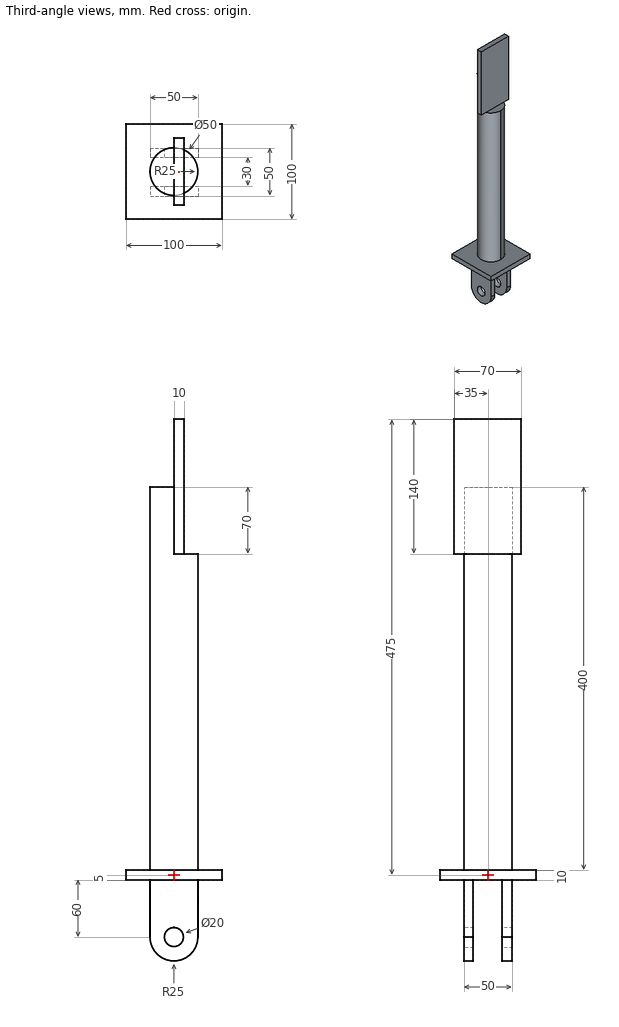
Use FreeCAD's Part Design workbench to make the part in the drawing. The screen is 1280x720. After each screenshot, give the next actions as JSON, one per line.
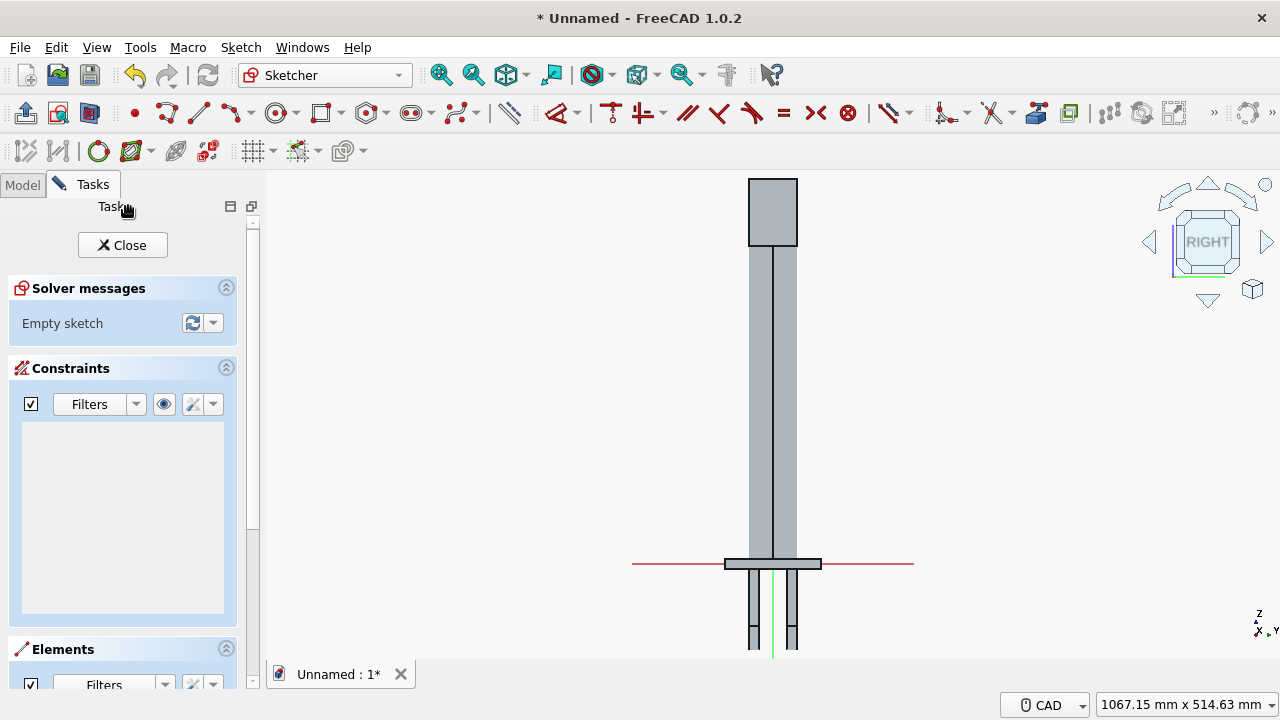
{"action": "key", "text": "q s"}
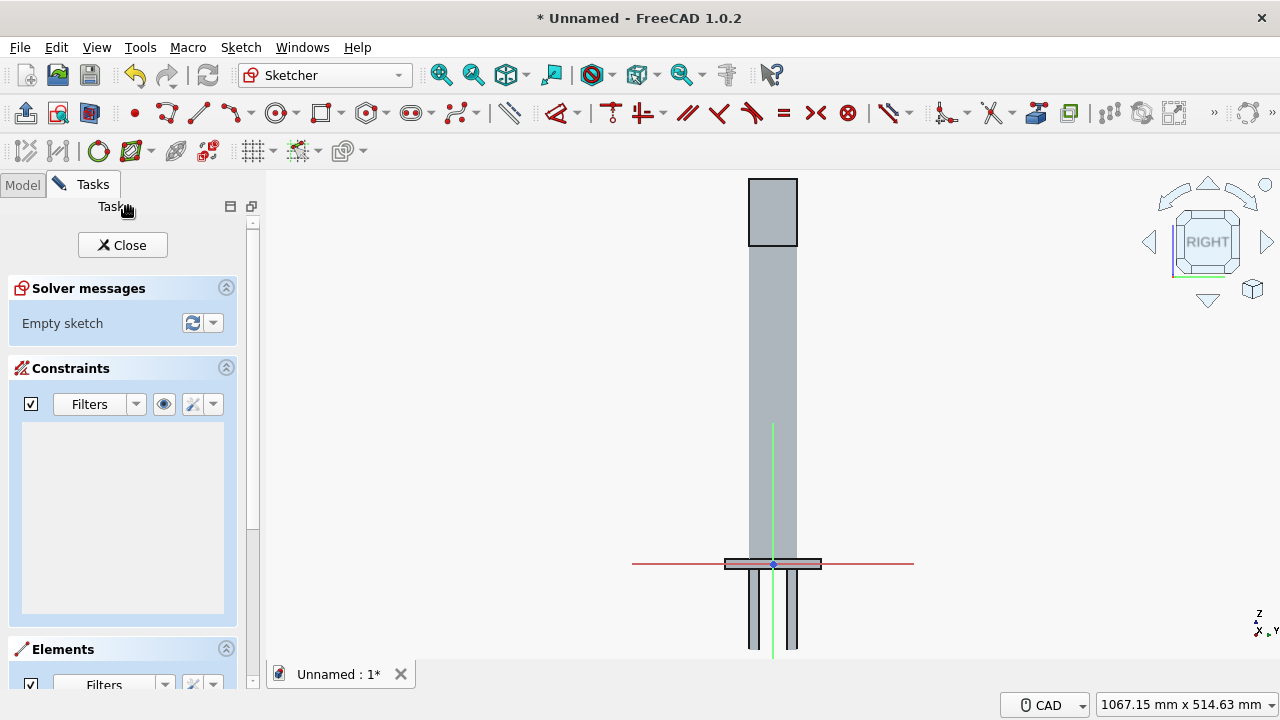
{"action": "scroll", "coordinate": [704, 414], "scroll_direction": "down", "scroll_amount": 5}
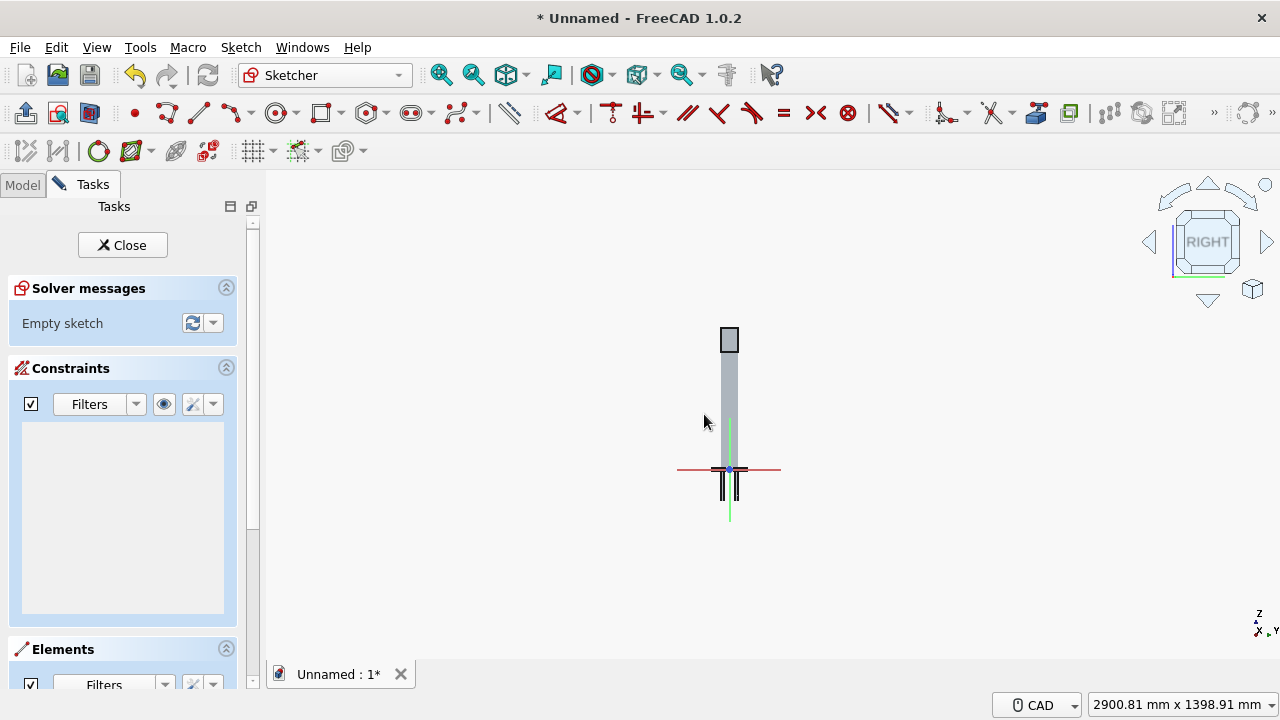
{"action": "scroll", "coordinate": [735, 311], "scroll_direction": "up", "scroll_amount": 9}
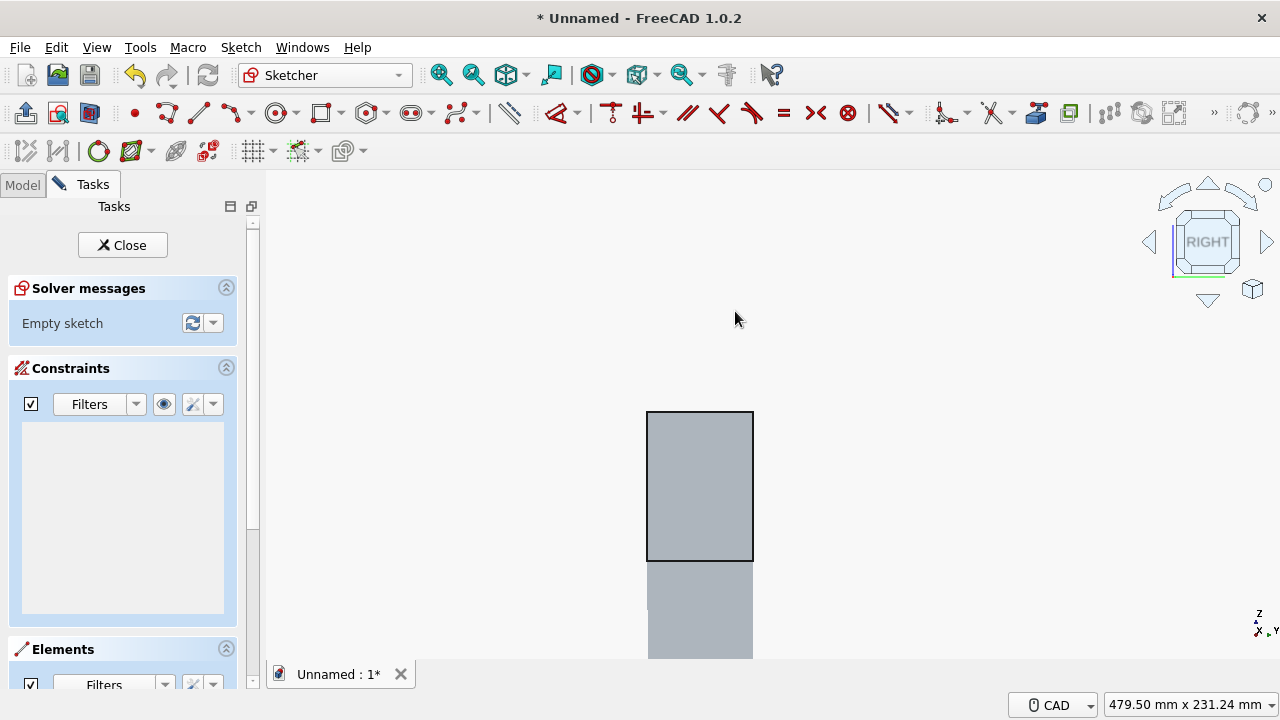
{"action": "key", "text": "g r"}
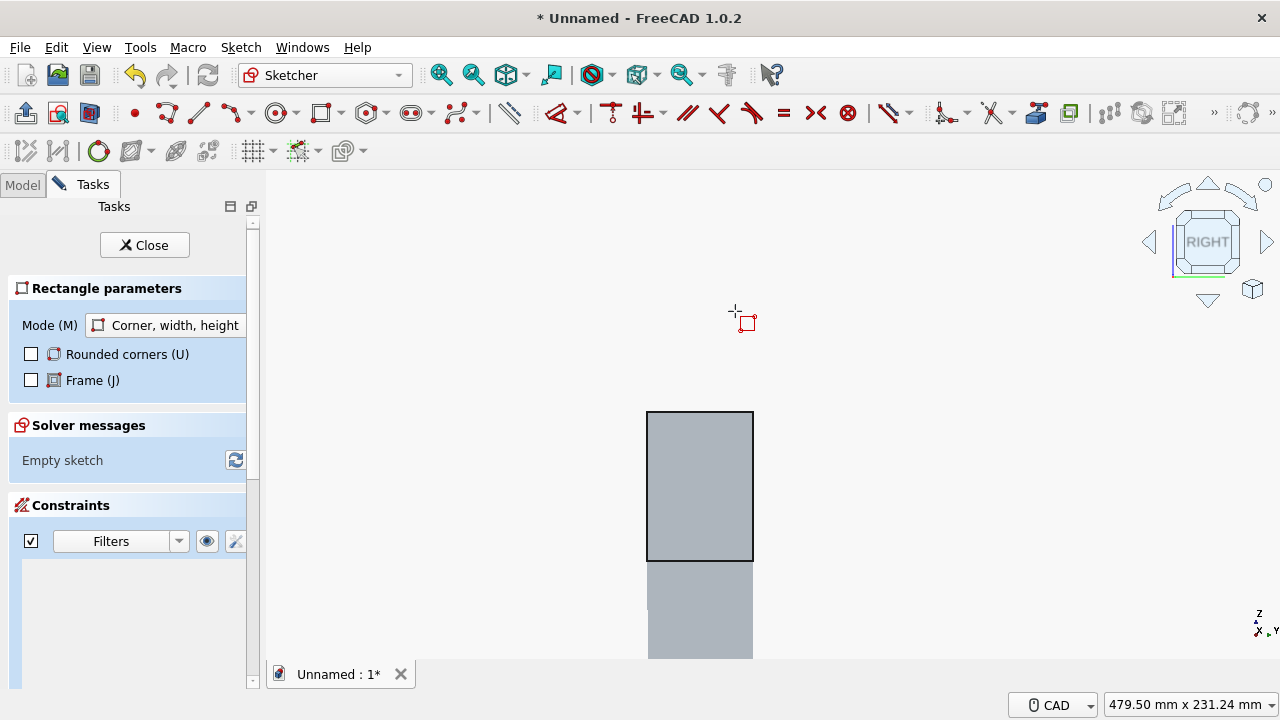
{"action": "left_click", "coordinate": [626, 264]}
{"action": "left_click", "coordinate": [774, 561]}
{"action": "key", "text": "Escape"}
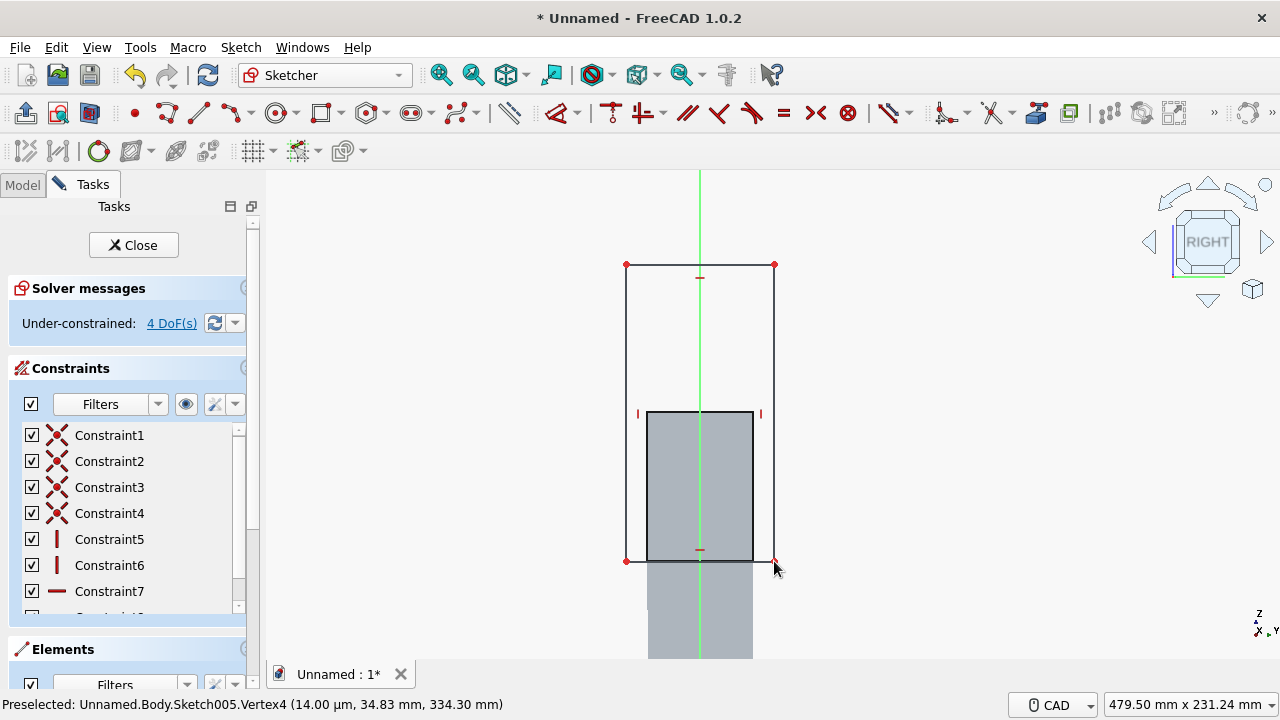
{"action": "left_click", "coordinate": [556, 114]}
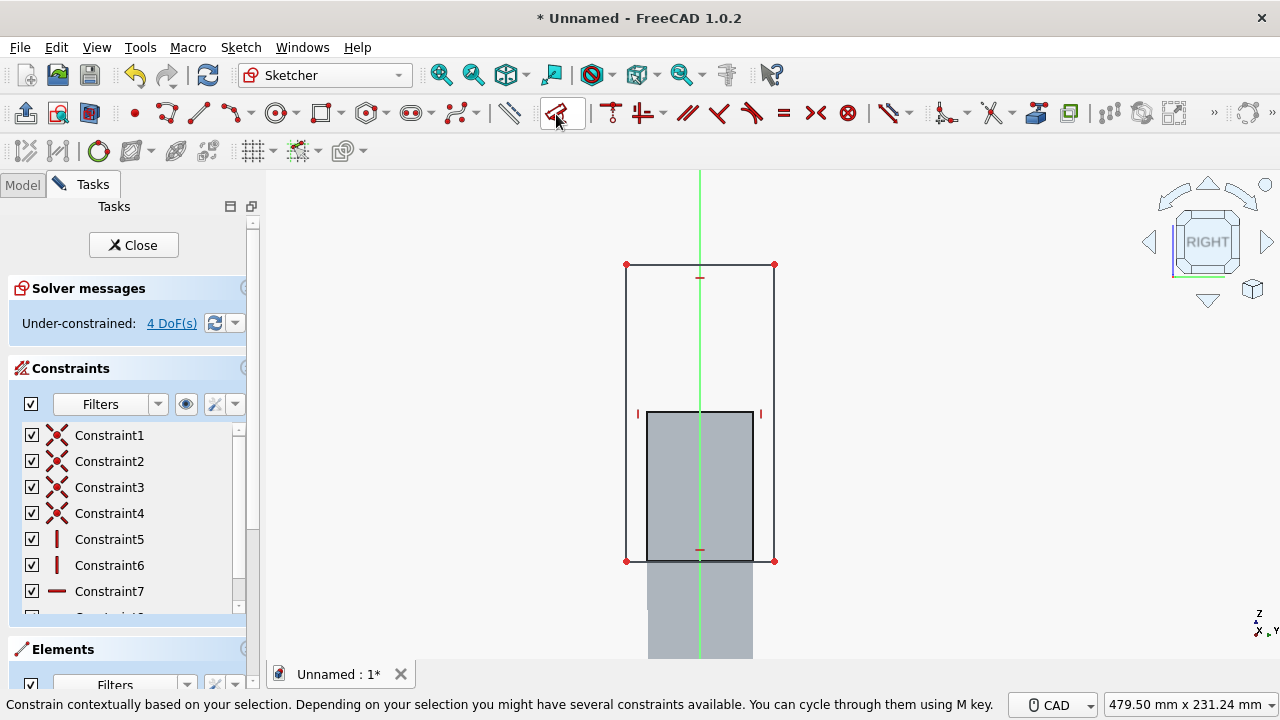
{"action": "left_click", "coordinate": [670, 562]}
{"action": "left_click", "coordinate": [666, 596]}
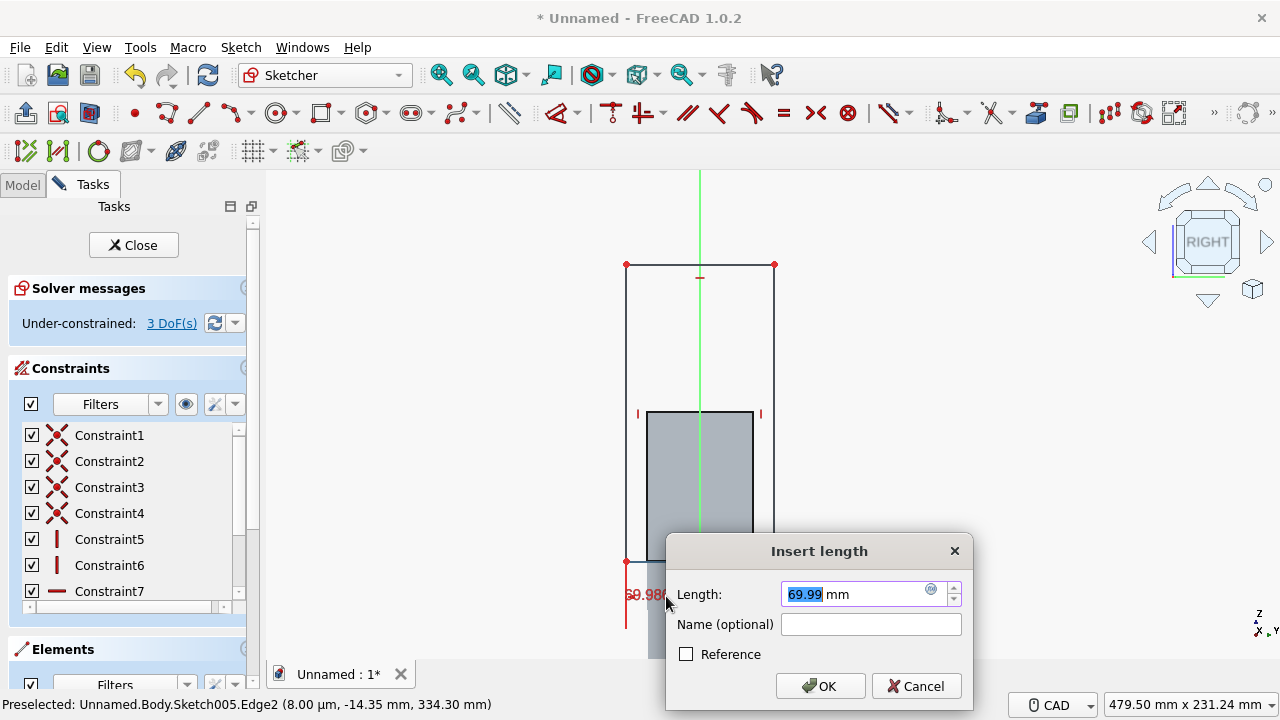
{"action": "type", "text": "70"}
{"action": "key", "text": "Return"}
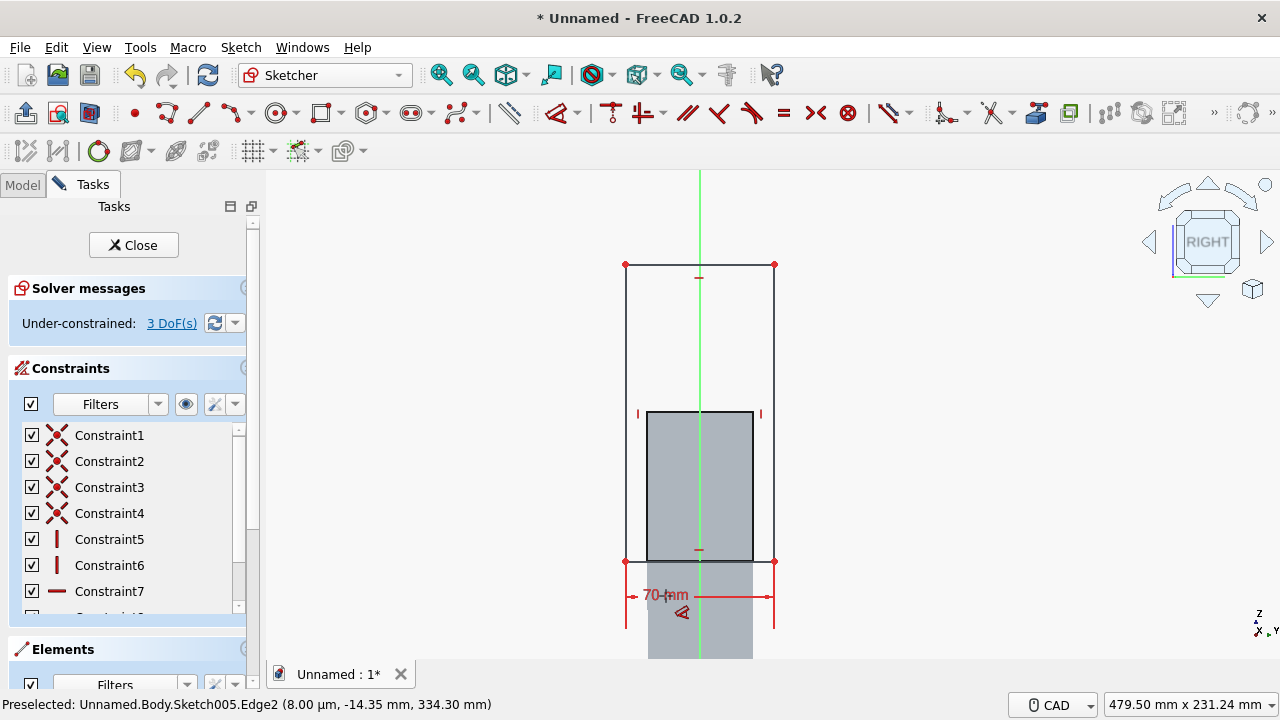
{"action": "left_click", "coordinate": [626, 354]}
{"action": "left_click", "coordinate": [592, 413]}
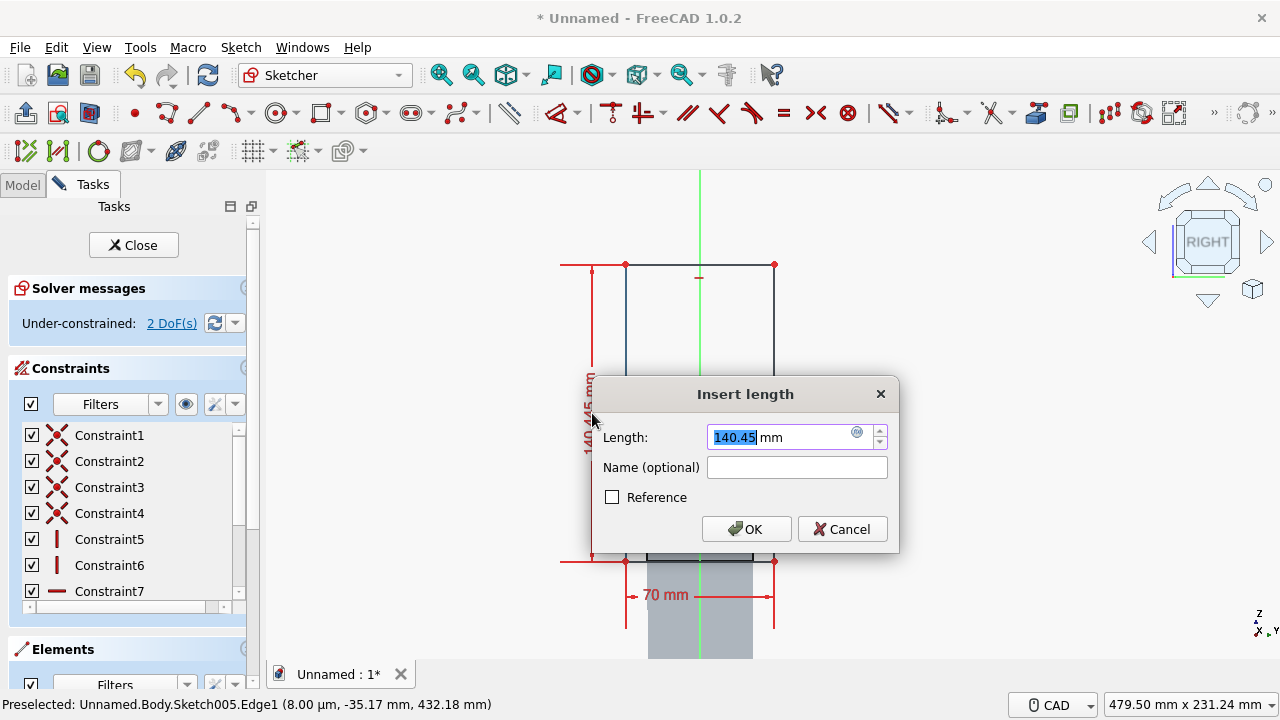
{"action": "type", "text": "140"}
{"action": "key", "text": "Return"}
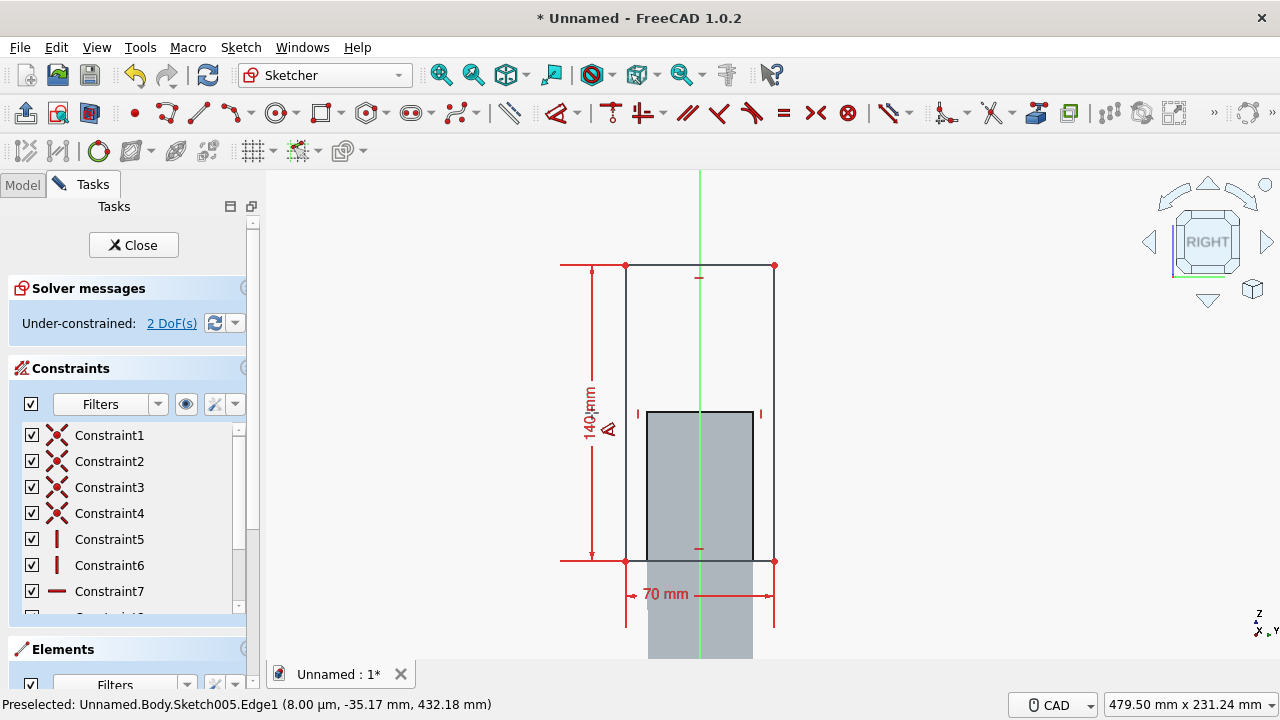
{"action": "left_click", "coordinate": [626, 265]}
{"action": "left_click", "coordinate": [663, 231]}